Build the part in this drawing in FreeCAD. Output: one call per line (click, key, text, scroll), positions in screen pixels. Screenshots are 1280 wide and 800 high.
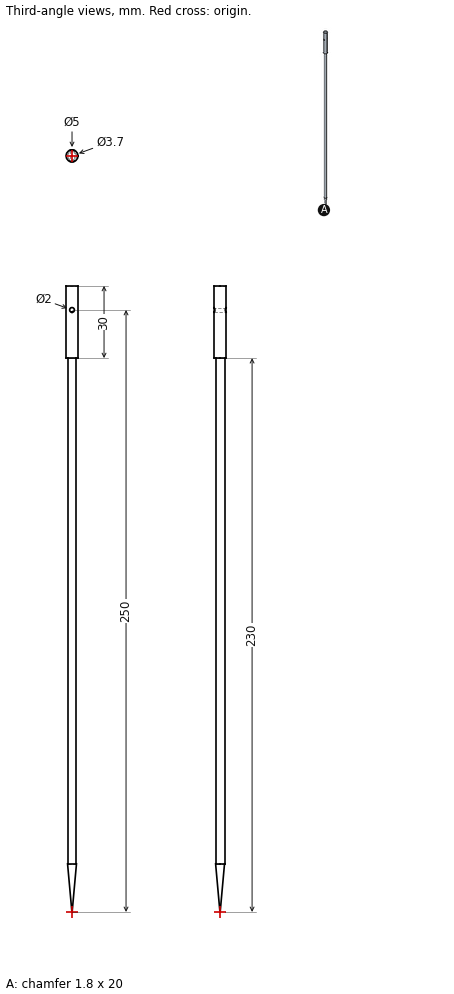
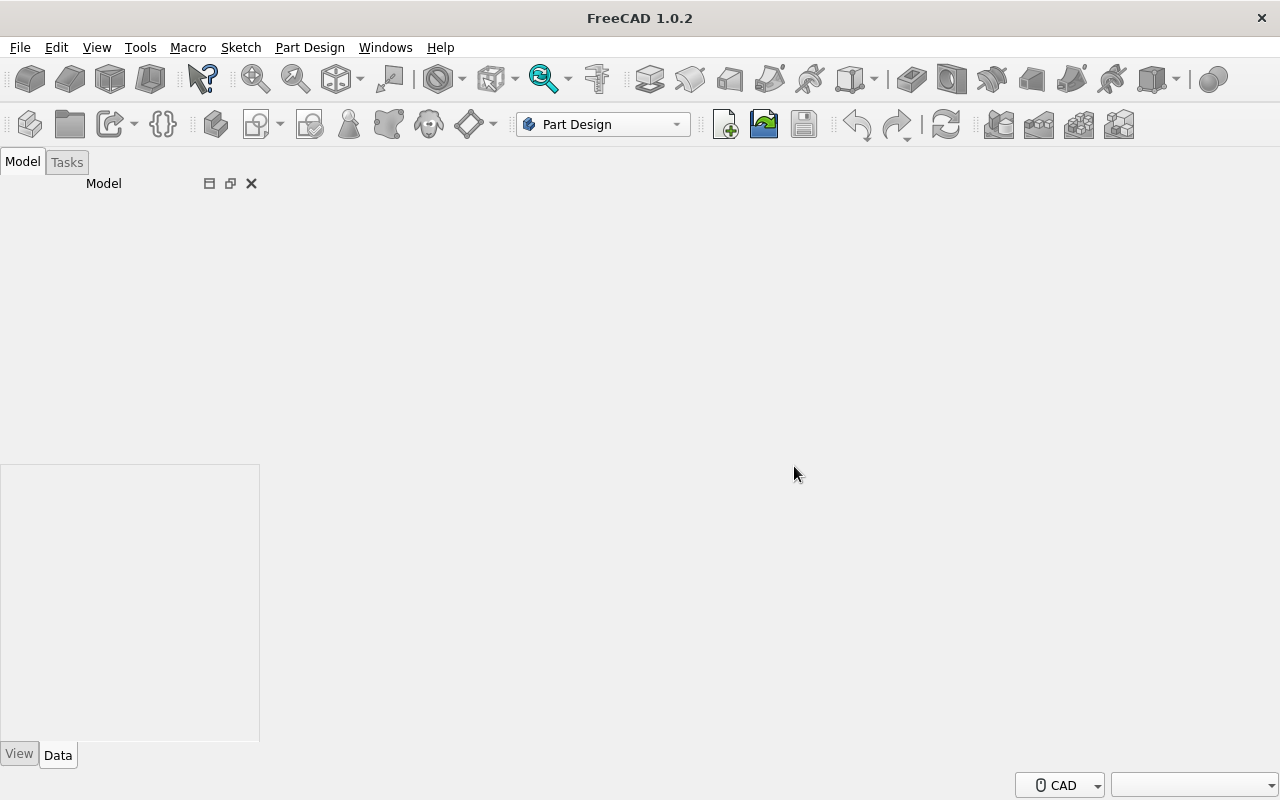
click(724, 124)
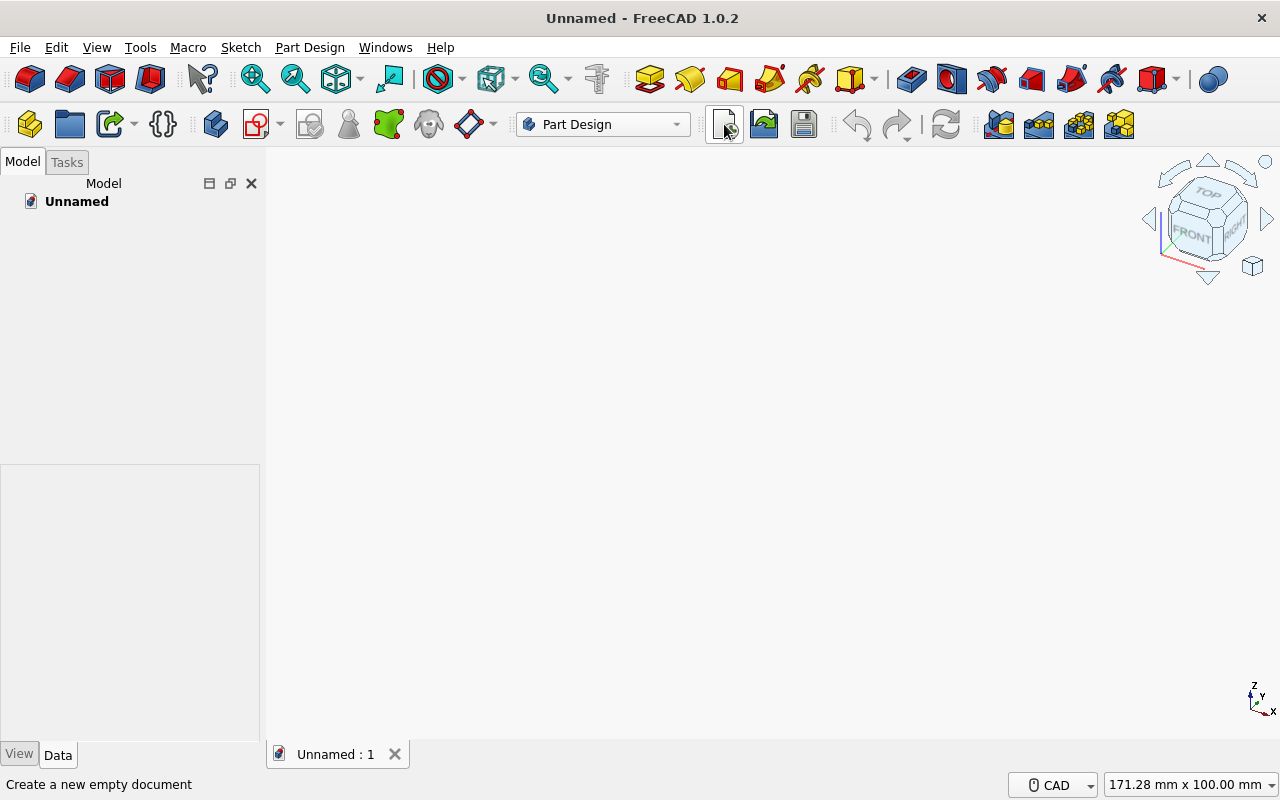
click(256, 124)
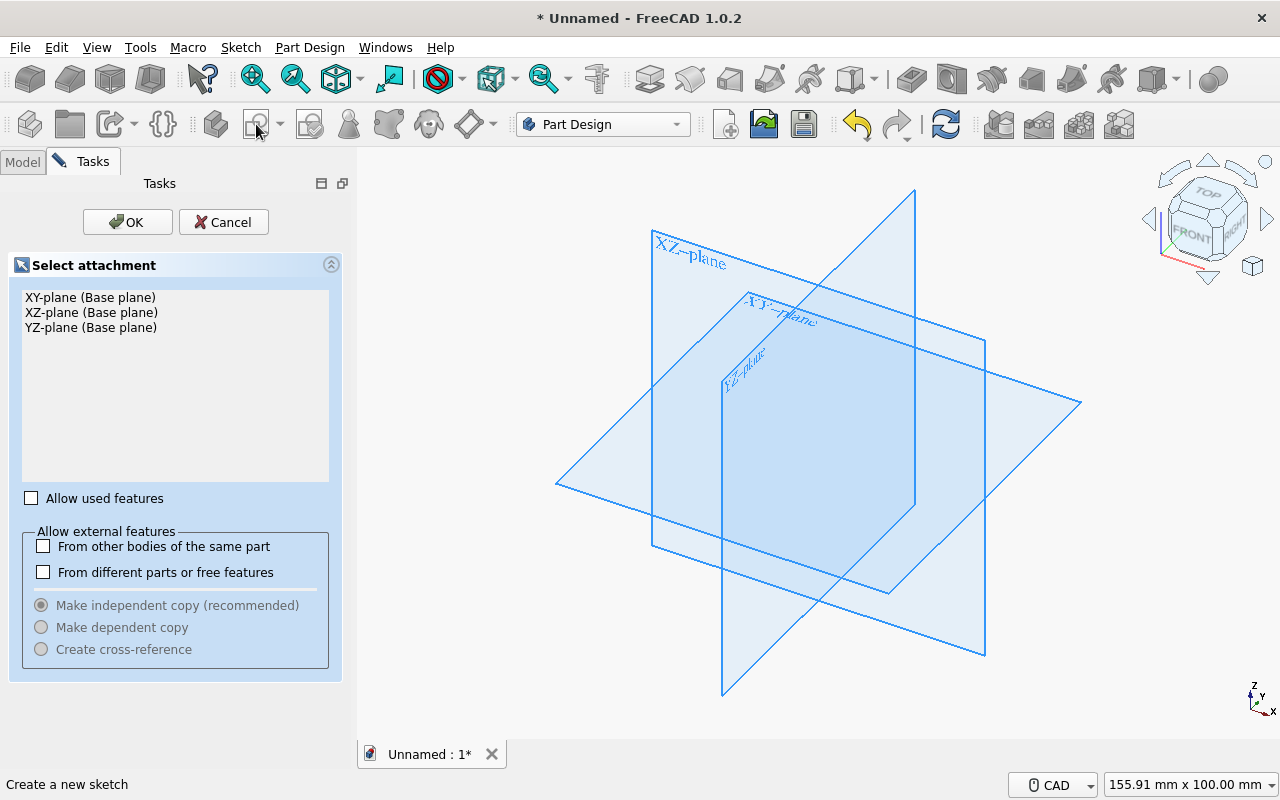
click(82, 298)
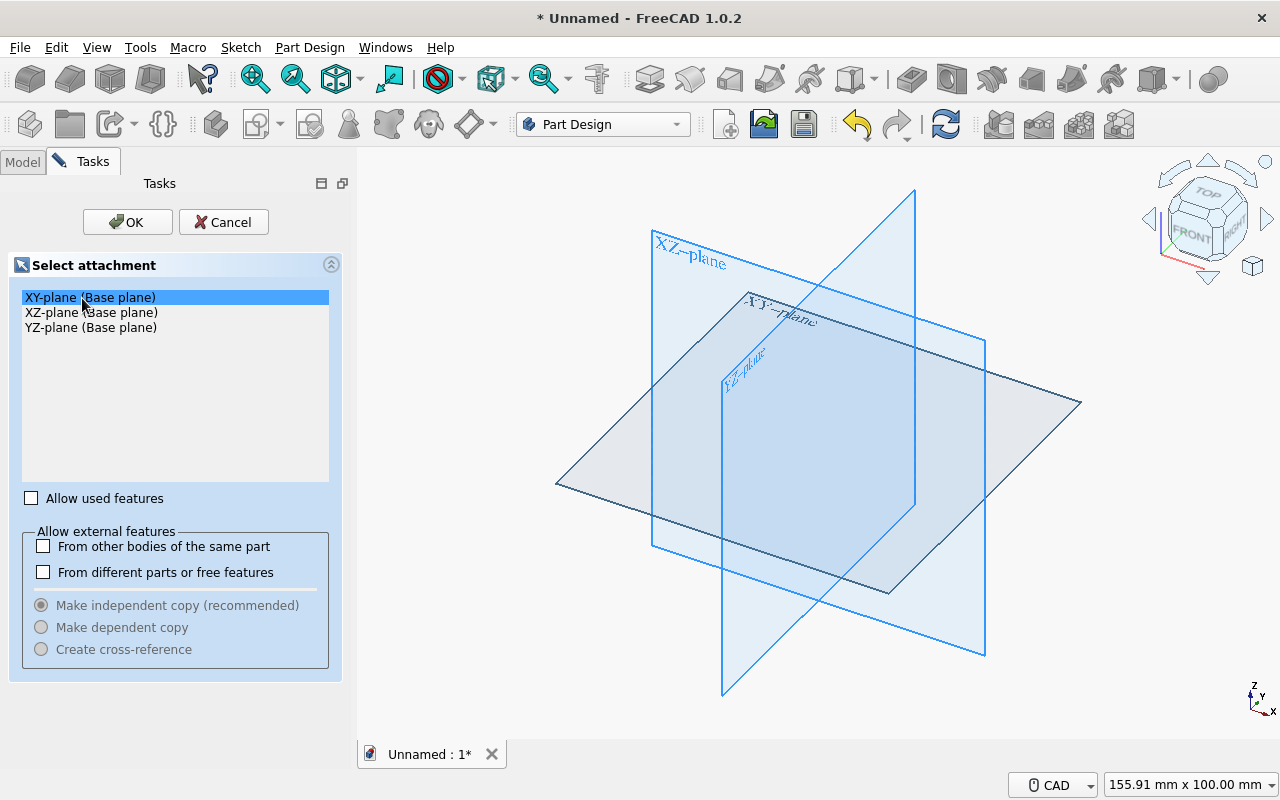
click(128, 222)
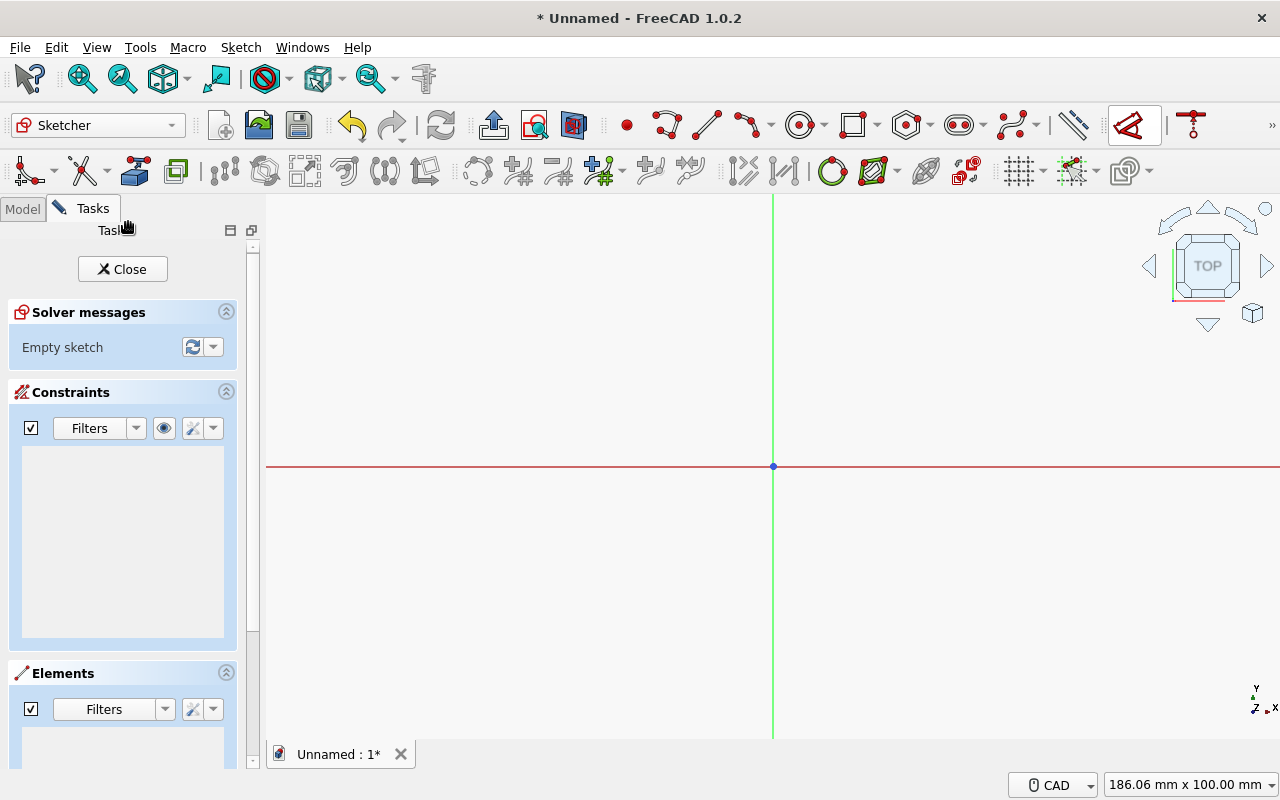
scroll(777, 466, up, 14)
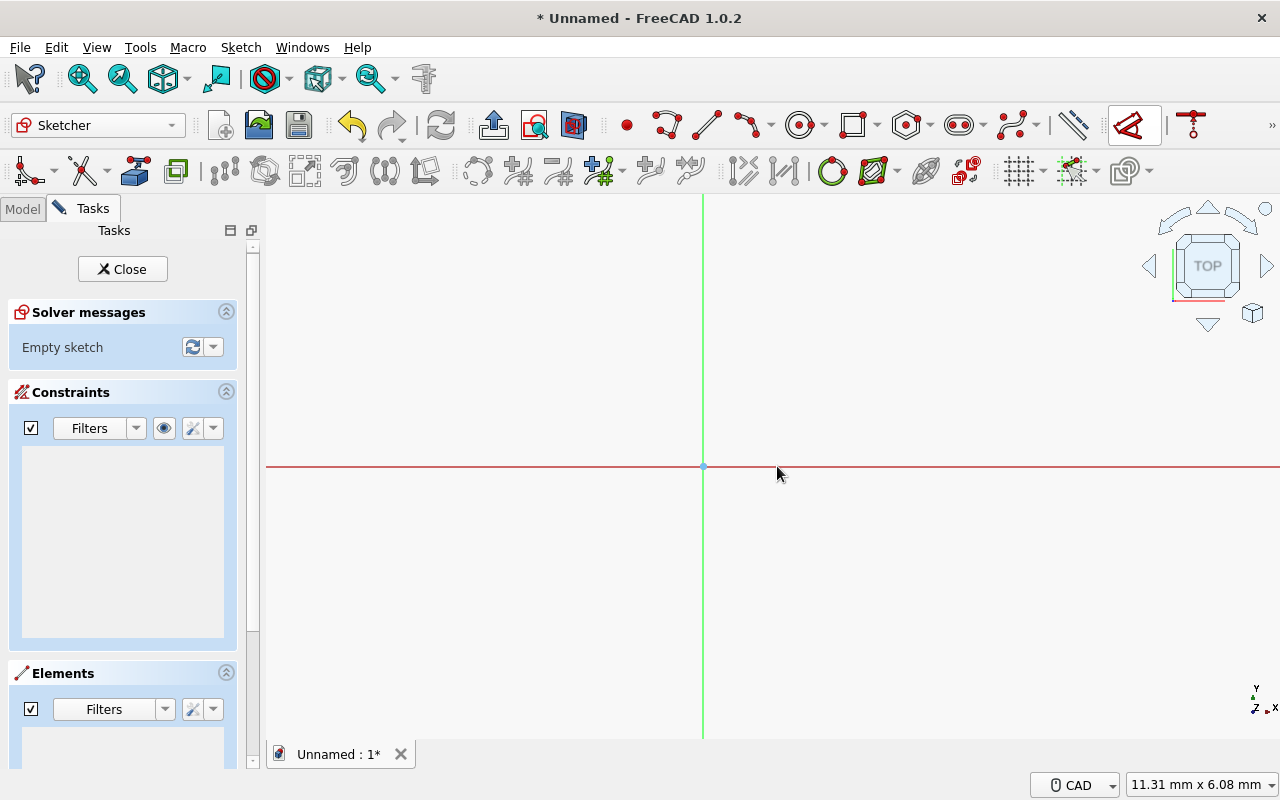
click(800, 126)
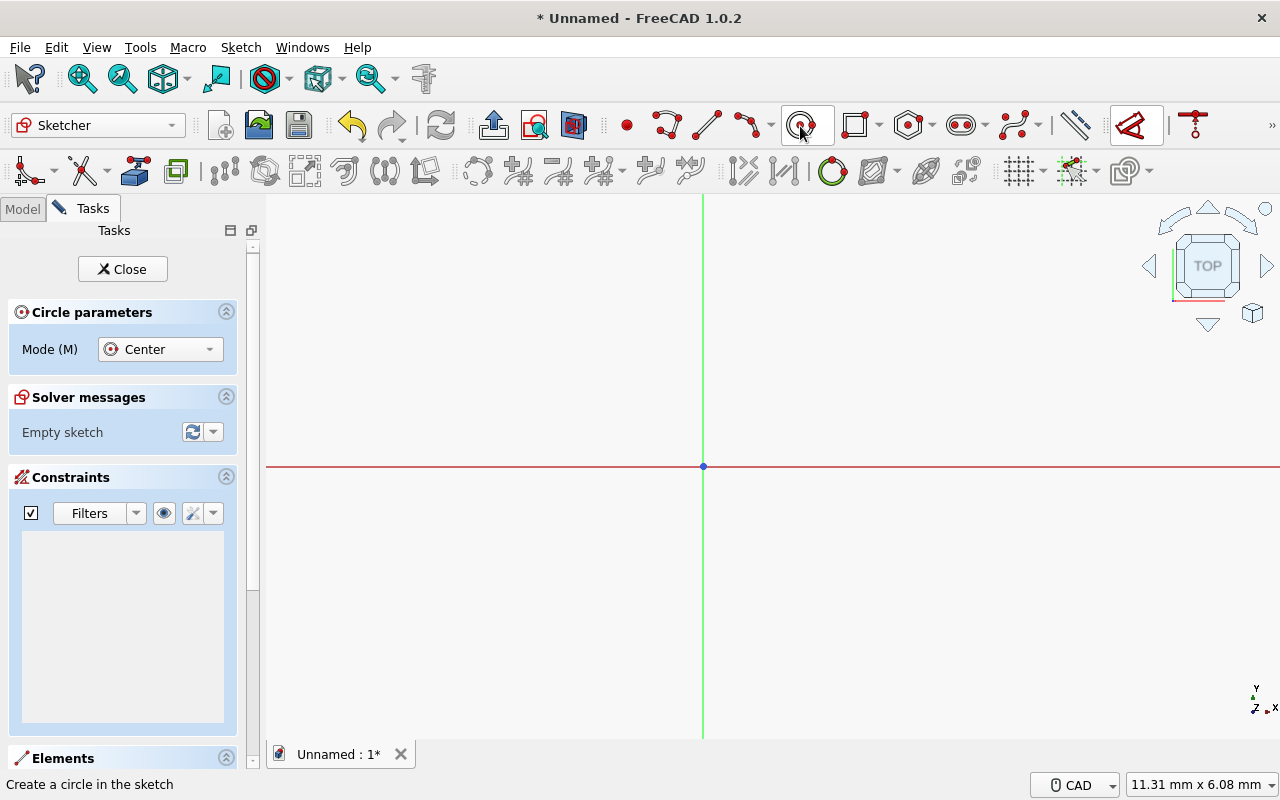
click(703, 466)
move(821, 349)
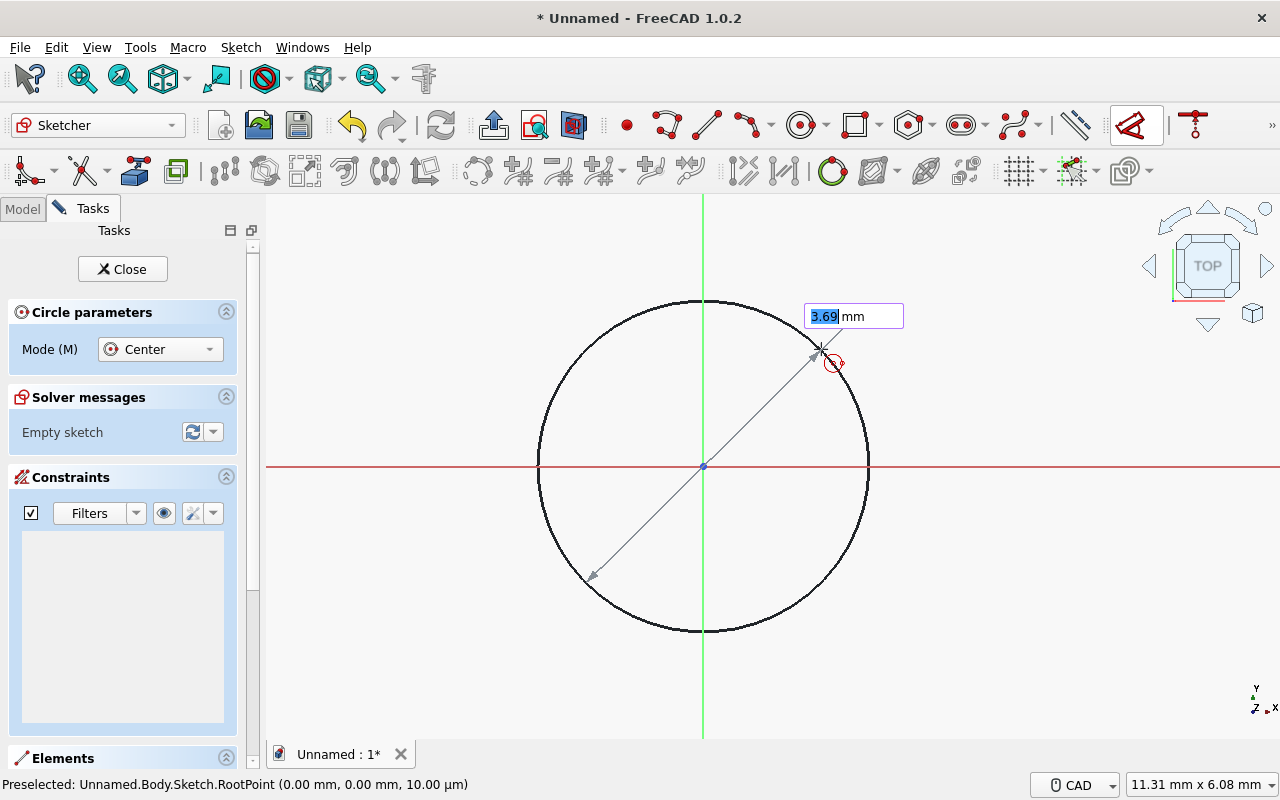
text(3.7)
key(Return)
key(Escape)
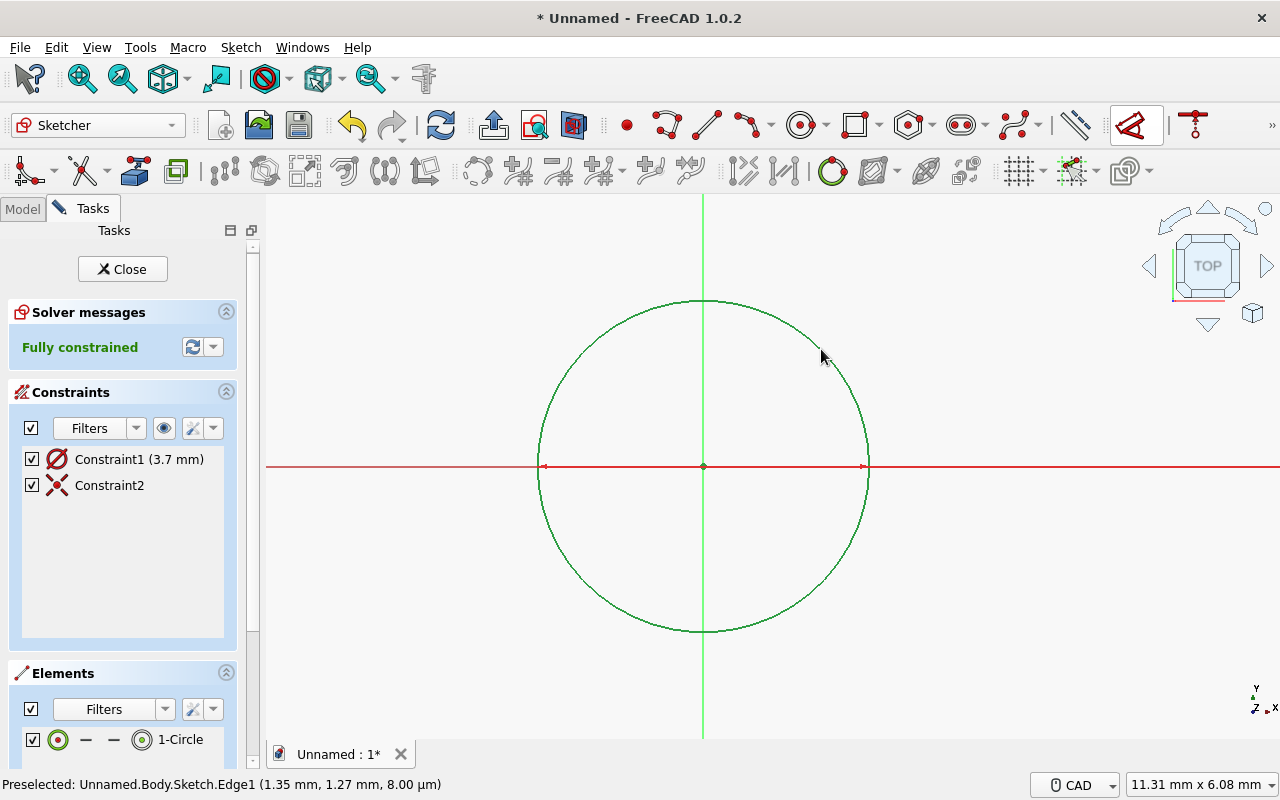
click(123, 269)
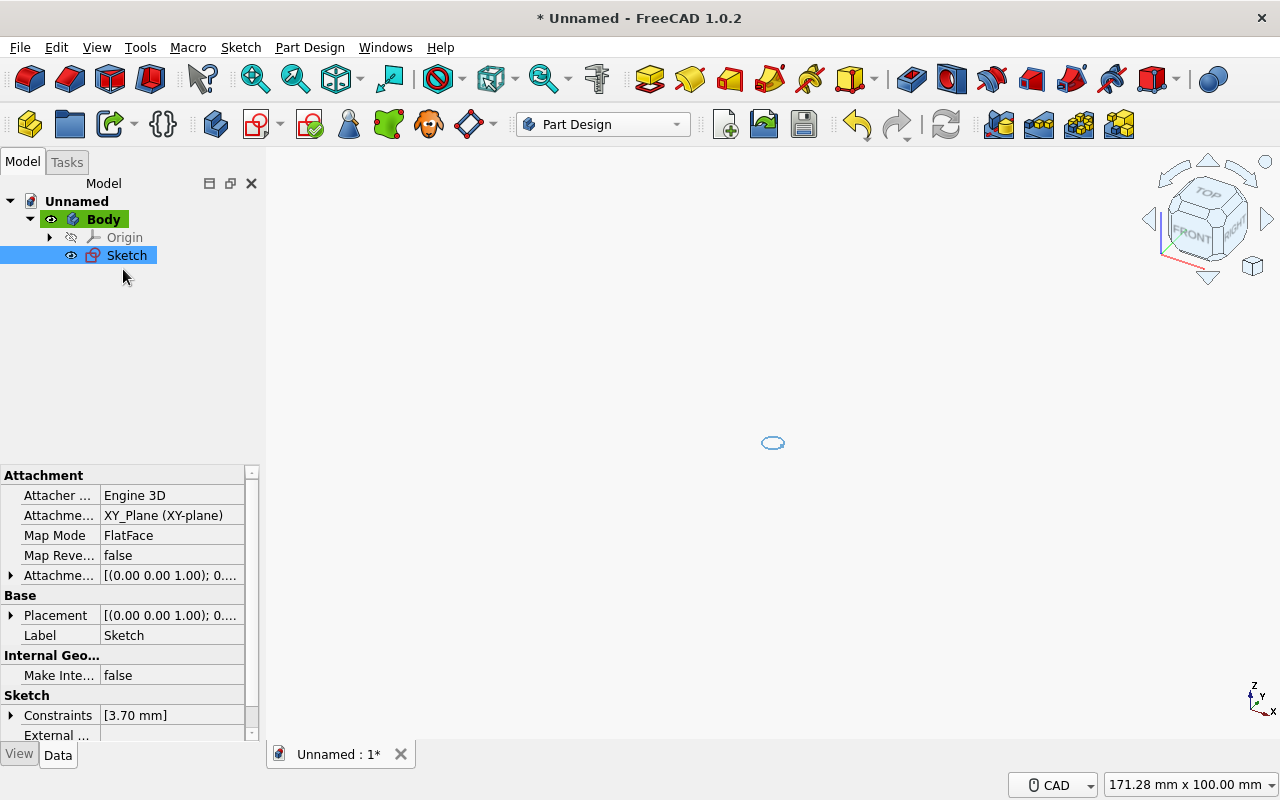
click(650, 80)